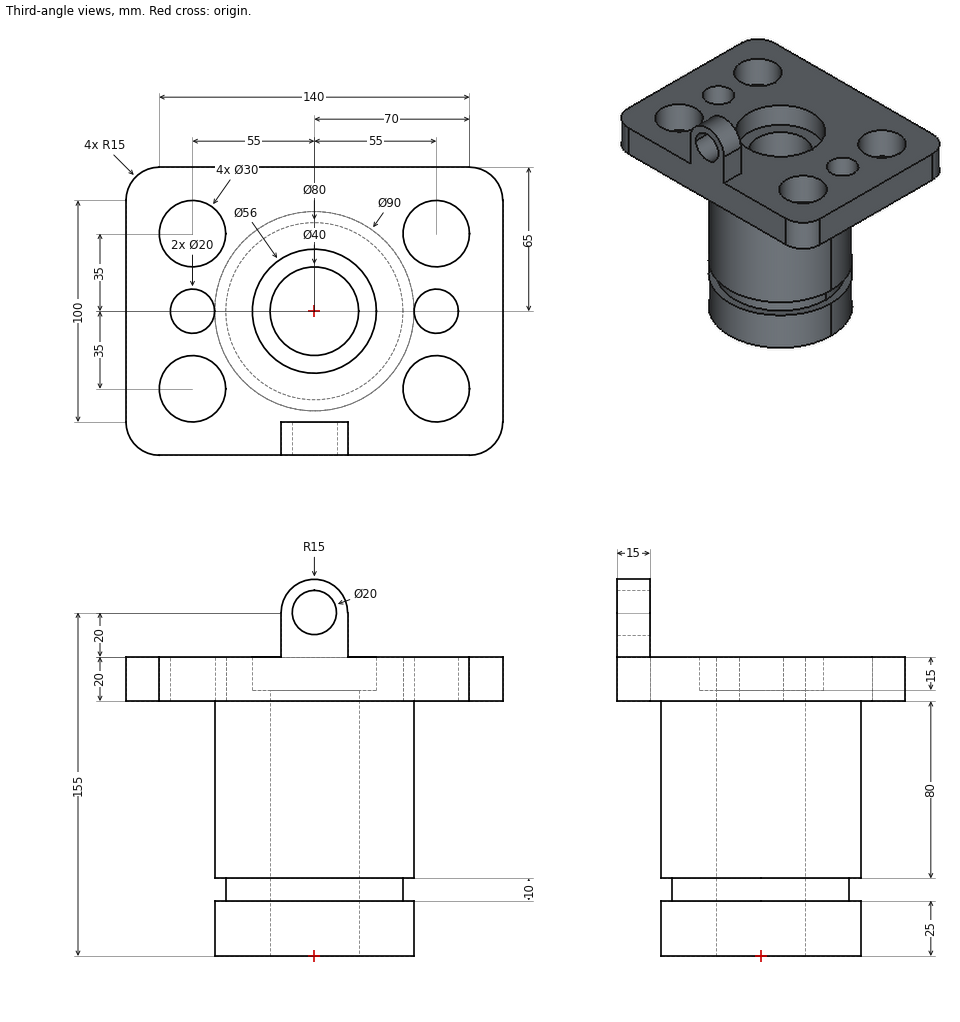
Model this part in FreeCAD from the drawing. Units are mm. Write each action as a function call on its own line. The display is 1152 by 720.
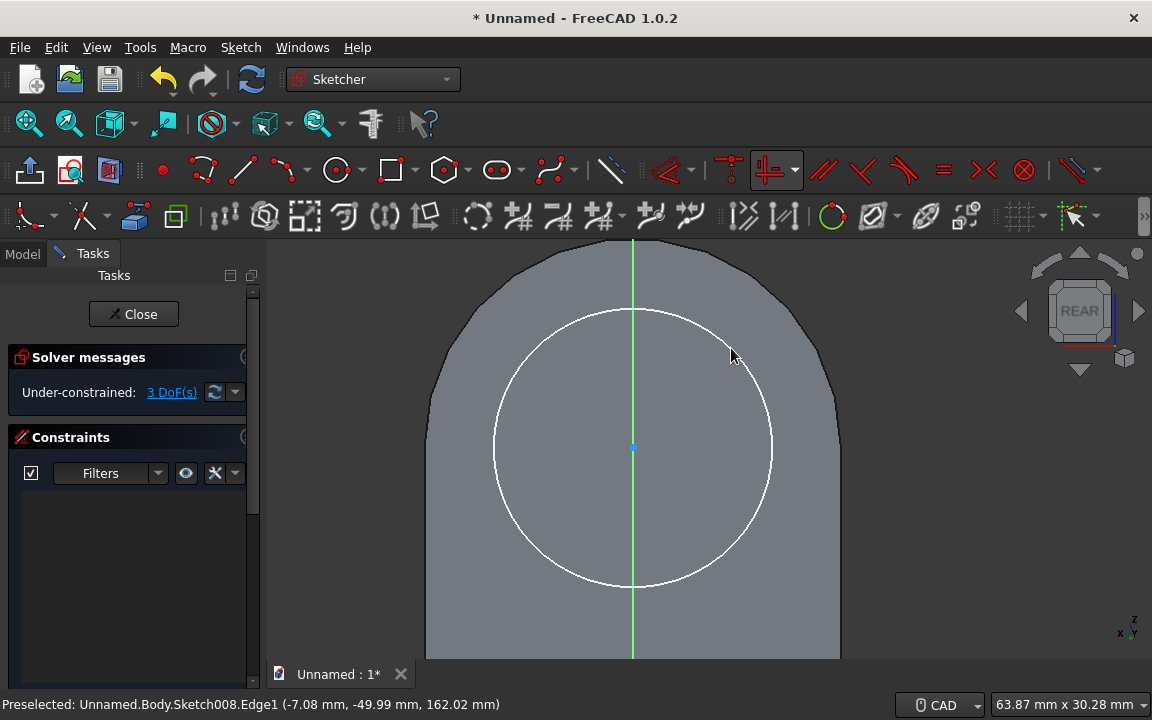
click(633, 448)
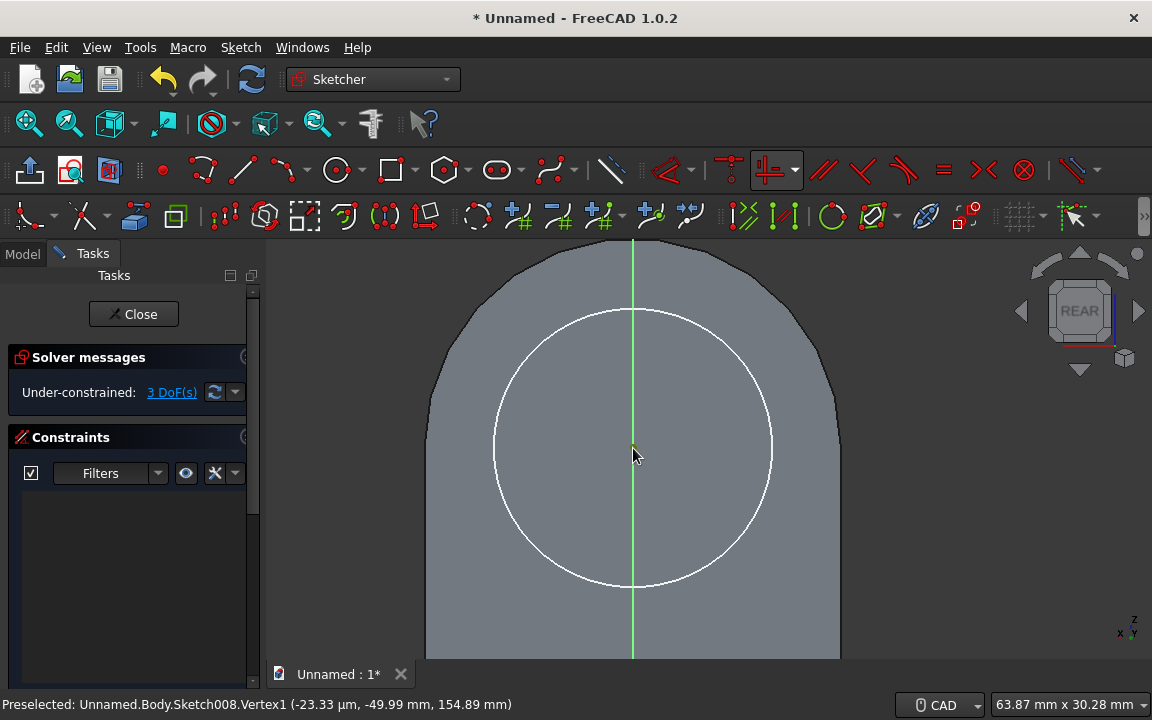
click(633, 553)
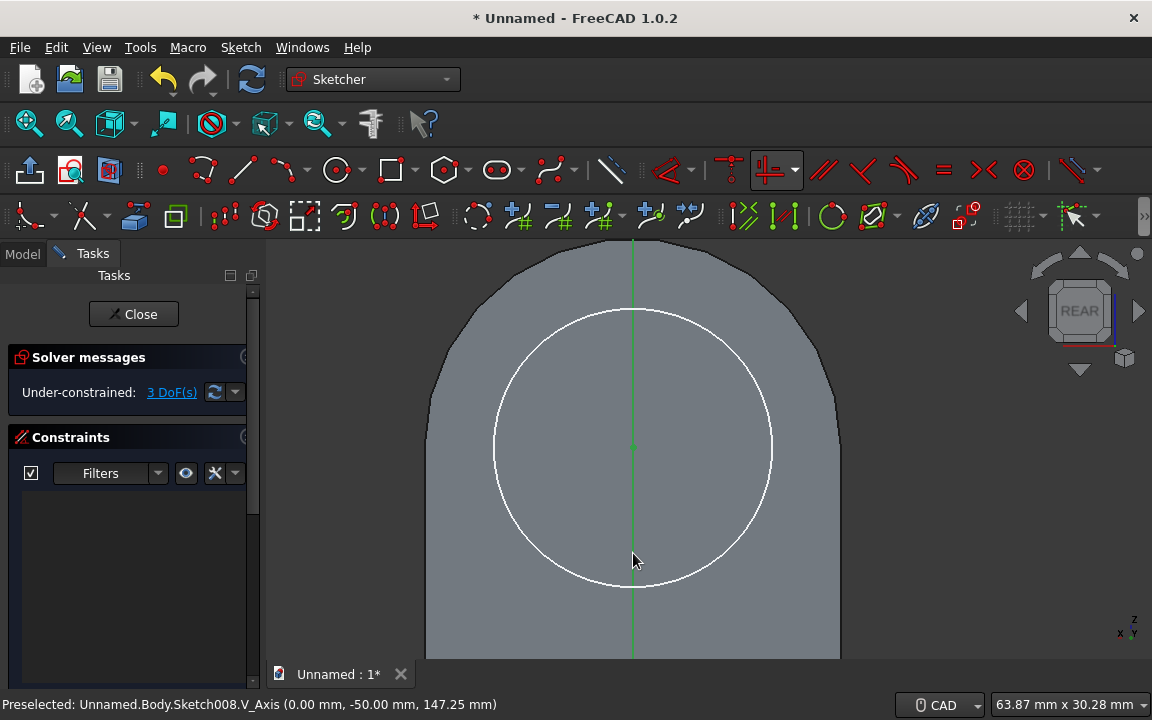
click(730, 170)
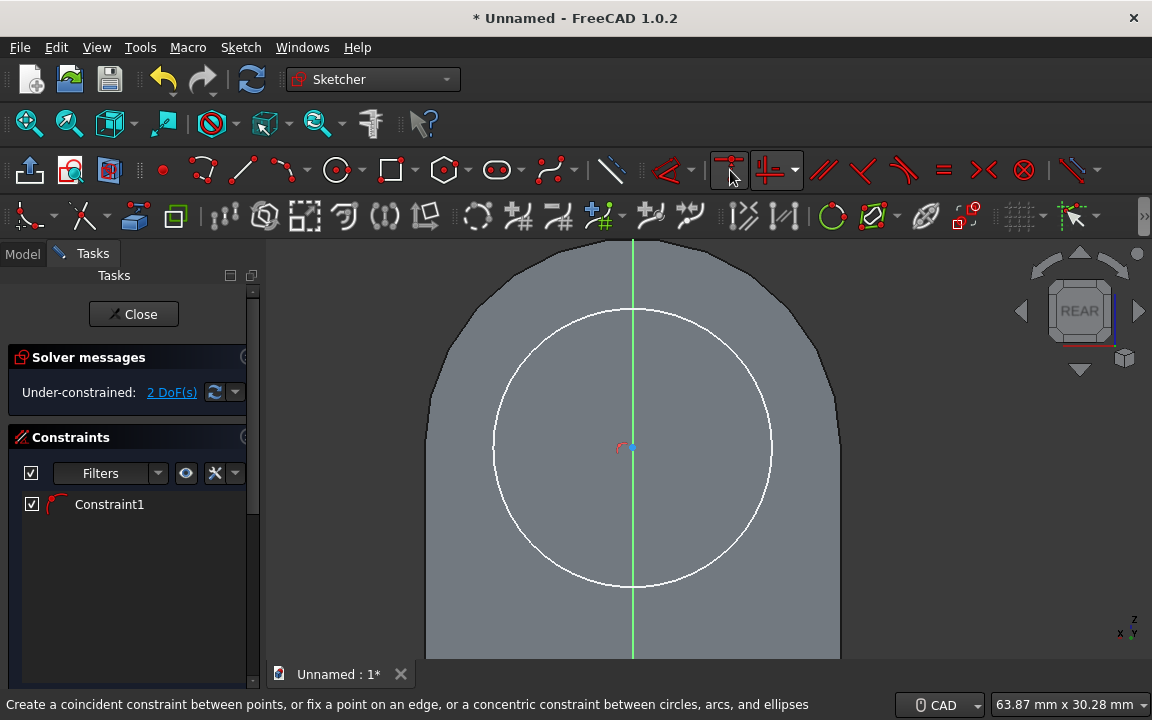
click(666, 170)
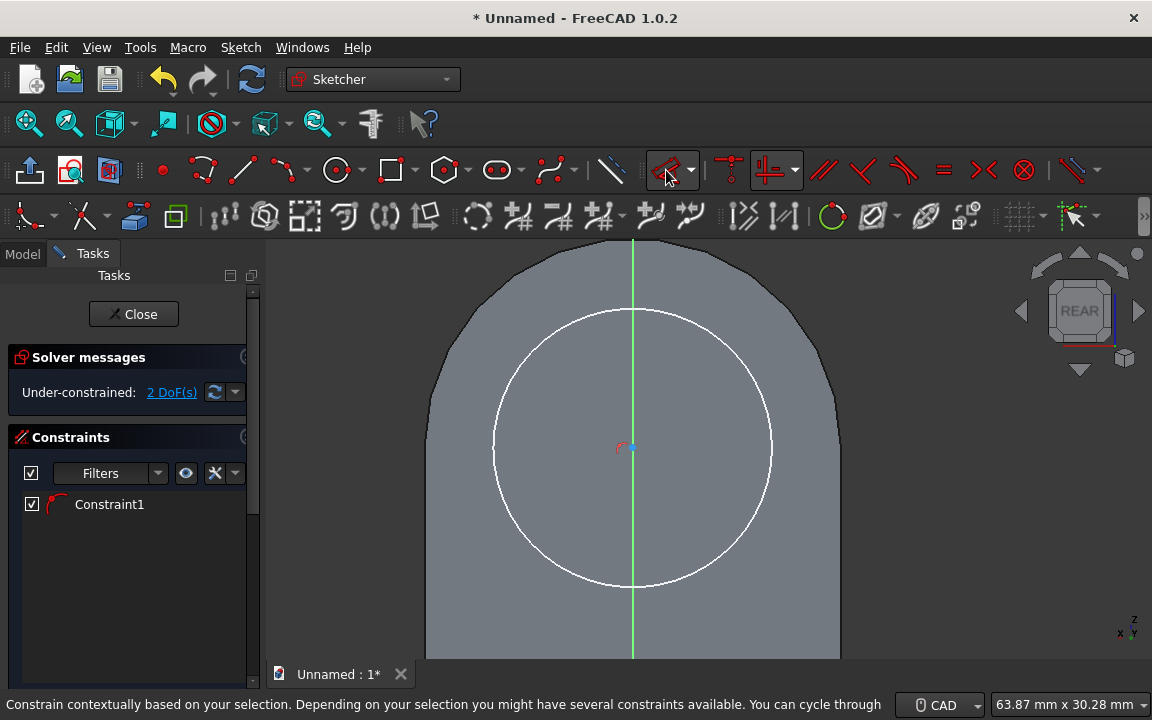
click(731, 349)
click(754, 326)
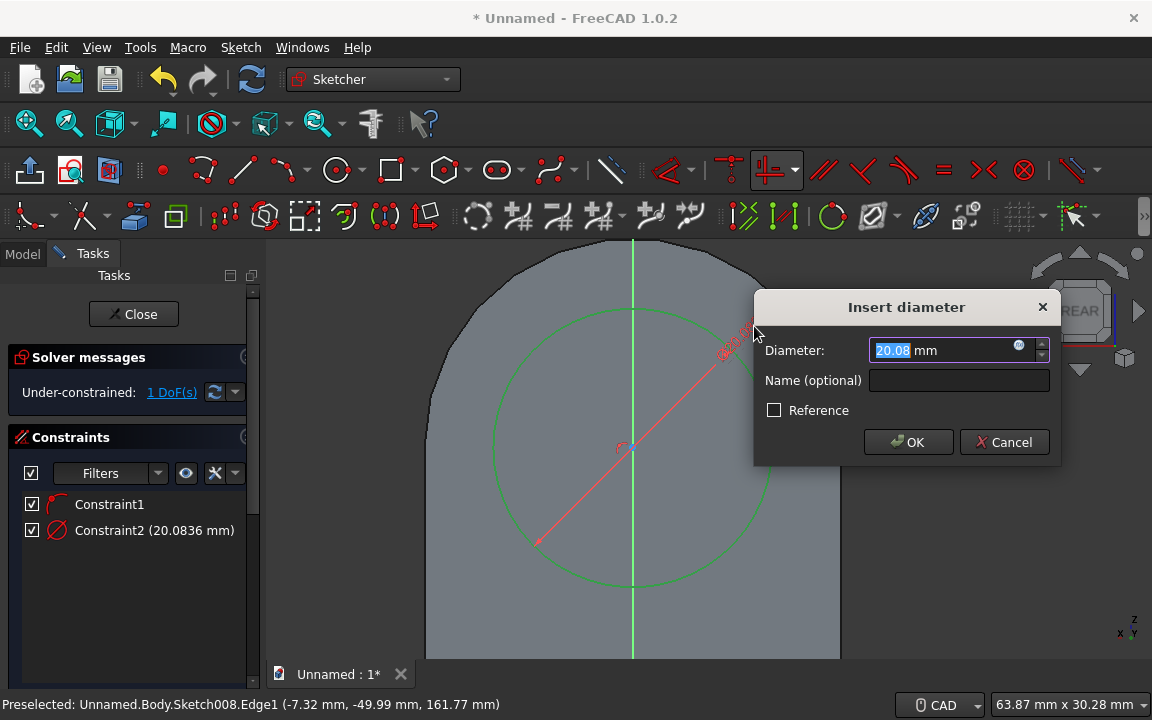
text(20)
key(Return)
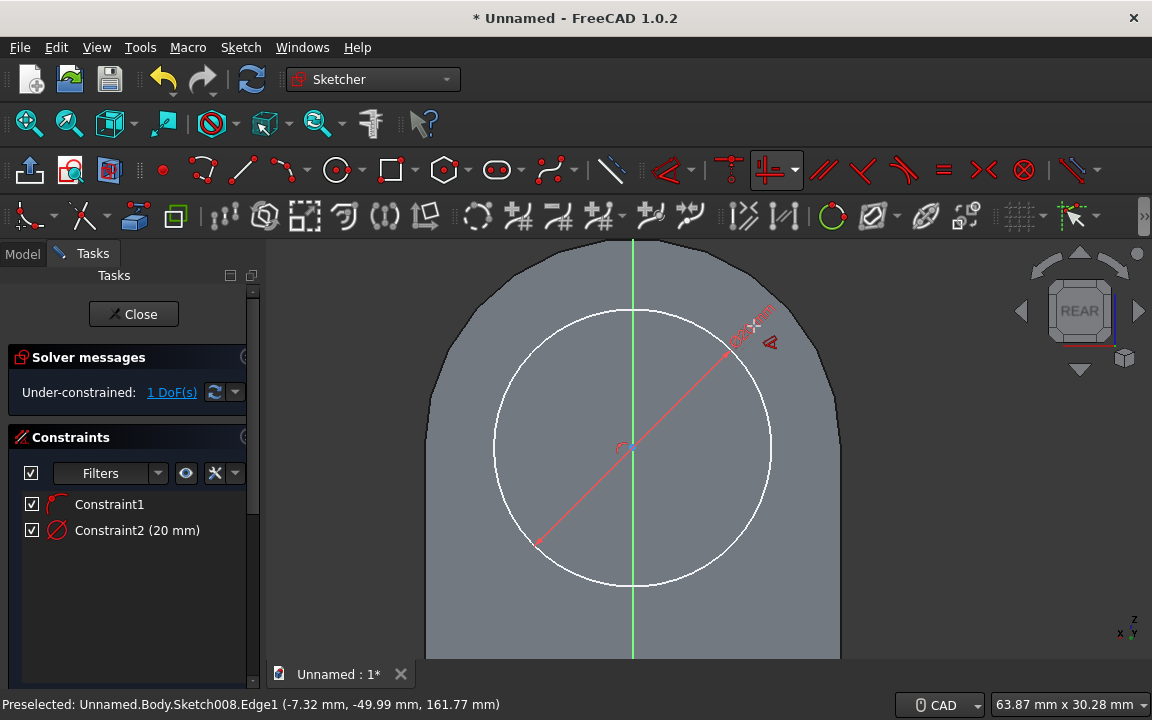
click(633, 448)
click(667, 540)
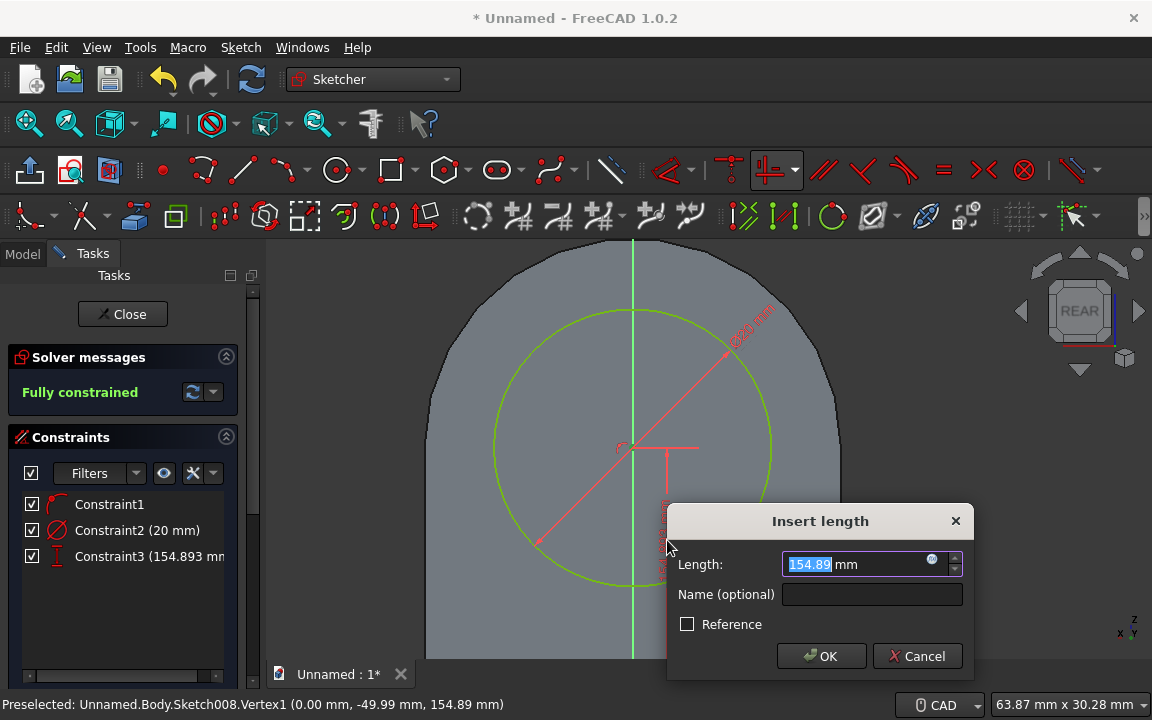
text(155)
key(Return)
key(Escape)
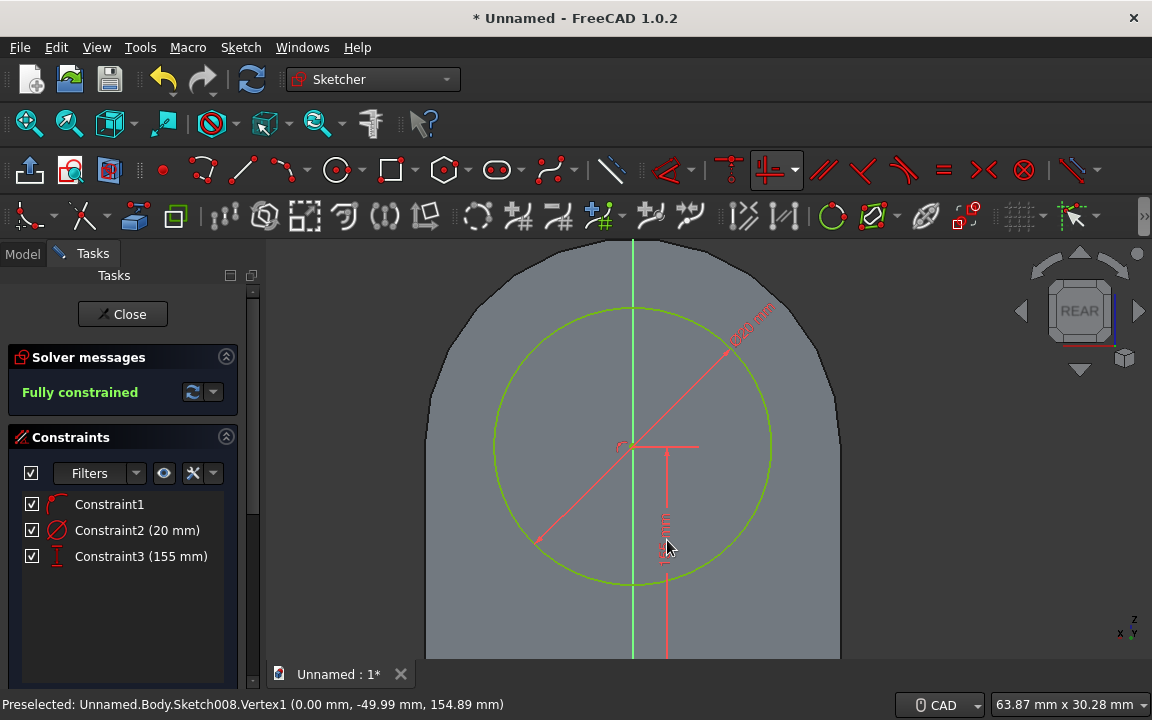
click(123, 314)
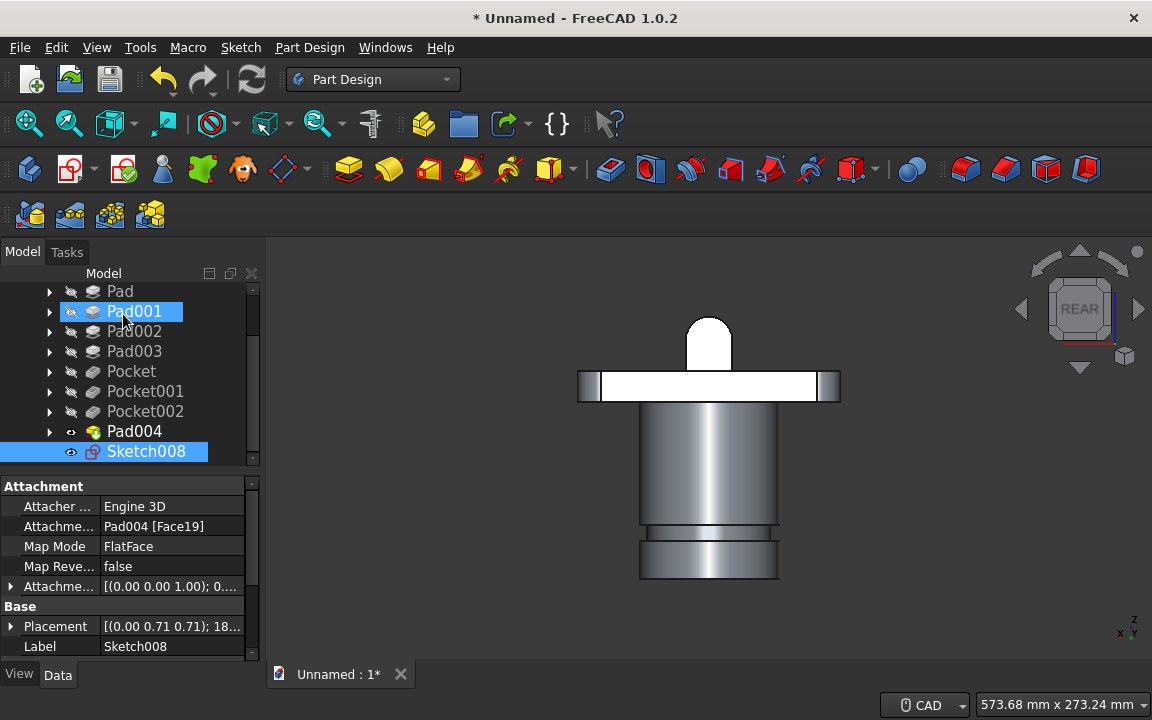
click(612, 170)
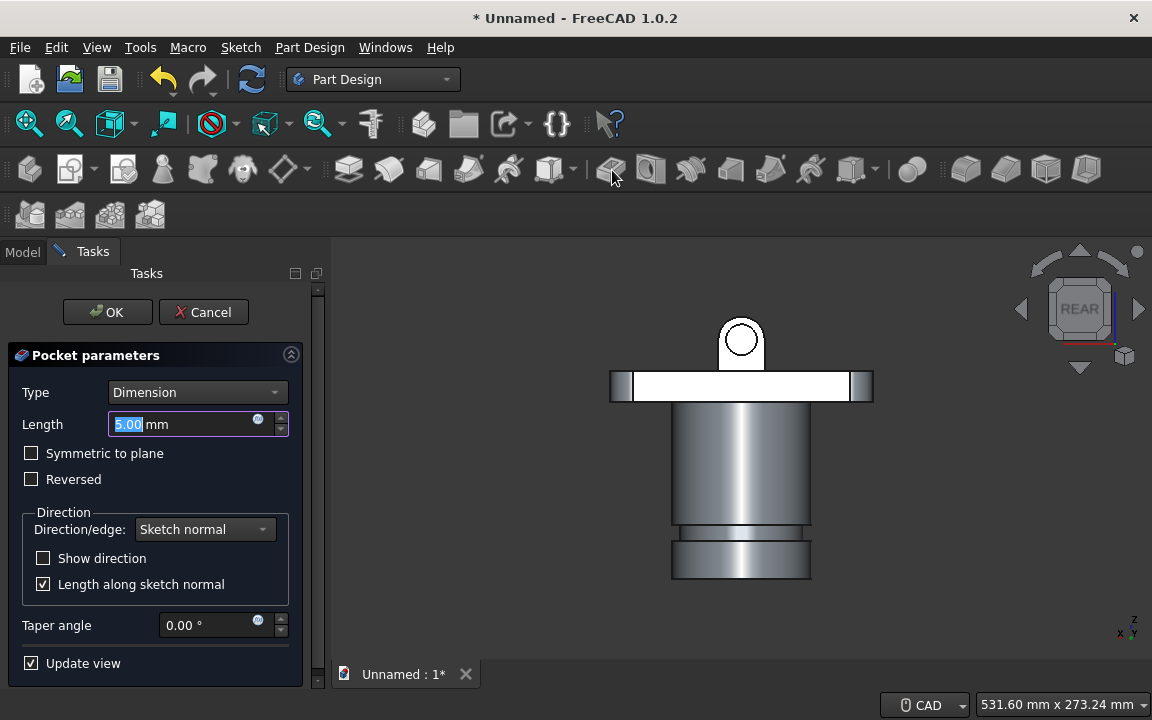
text(15)
key(Tab)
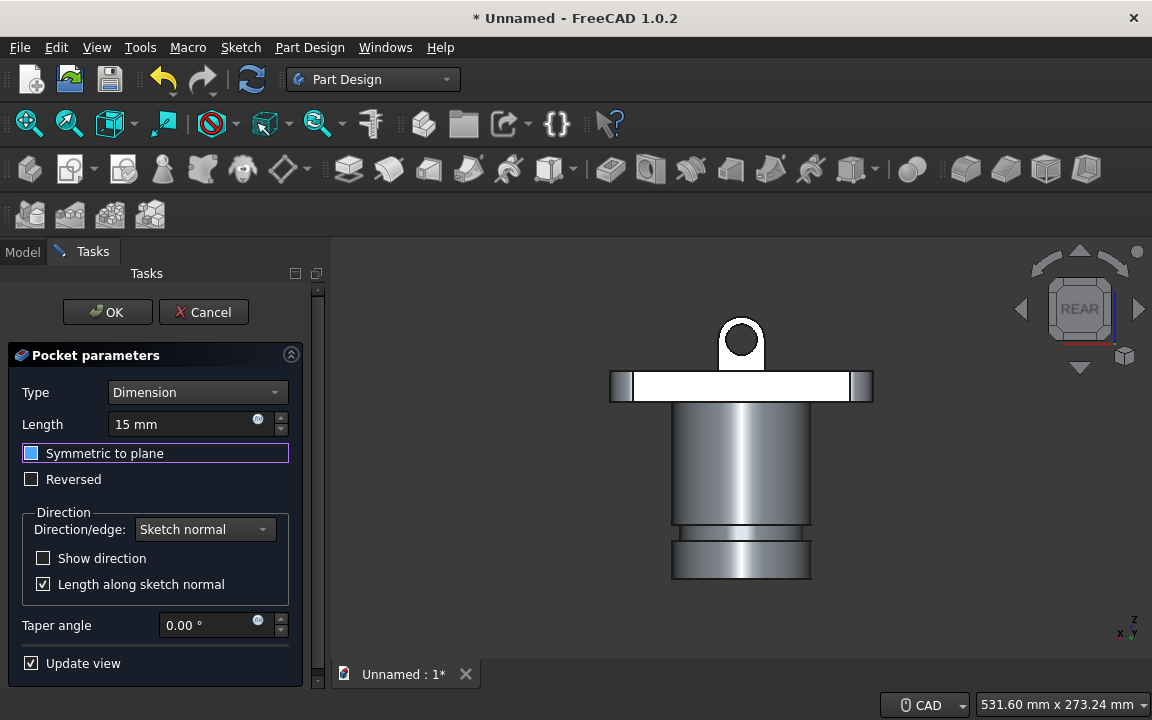
click(108, 312)